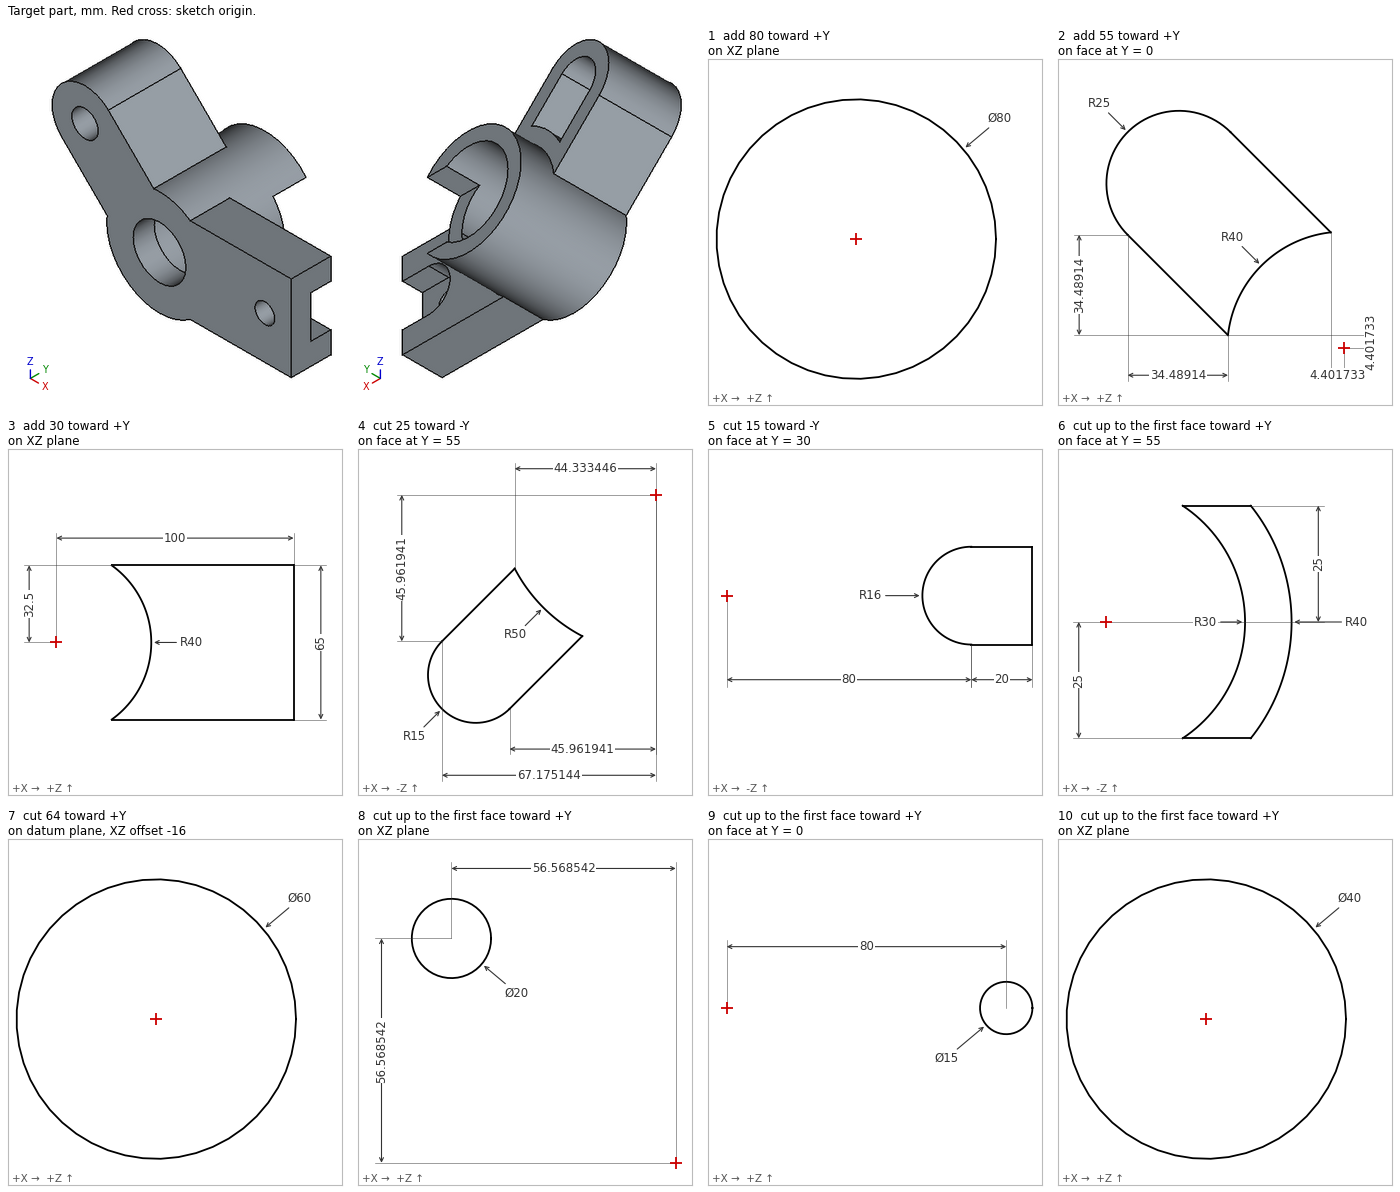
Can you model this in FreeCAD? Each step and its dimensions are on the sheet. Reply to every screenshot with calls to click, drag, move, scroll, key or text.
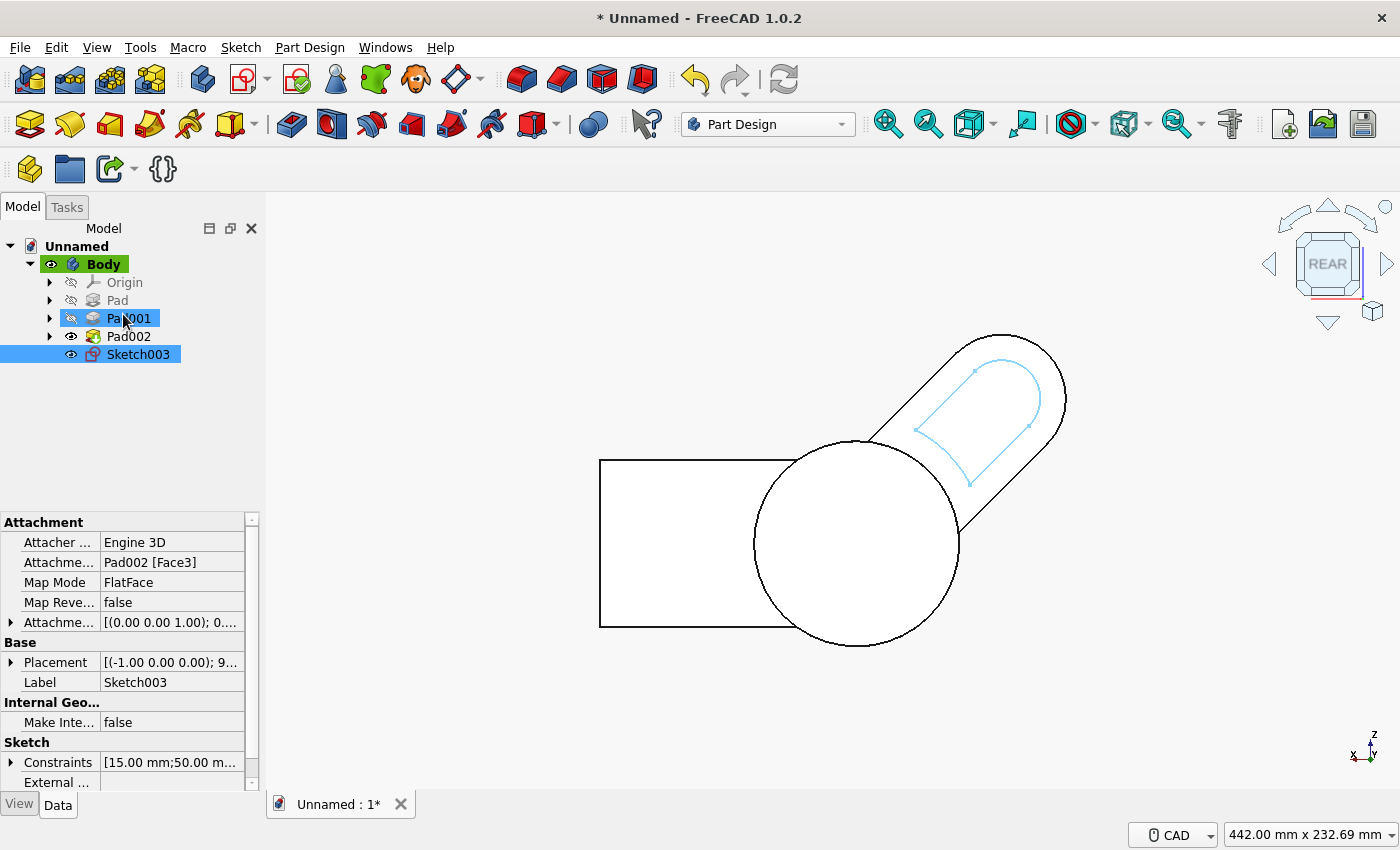
click(292, 124)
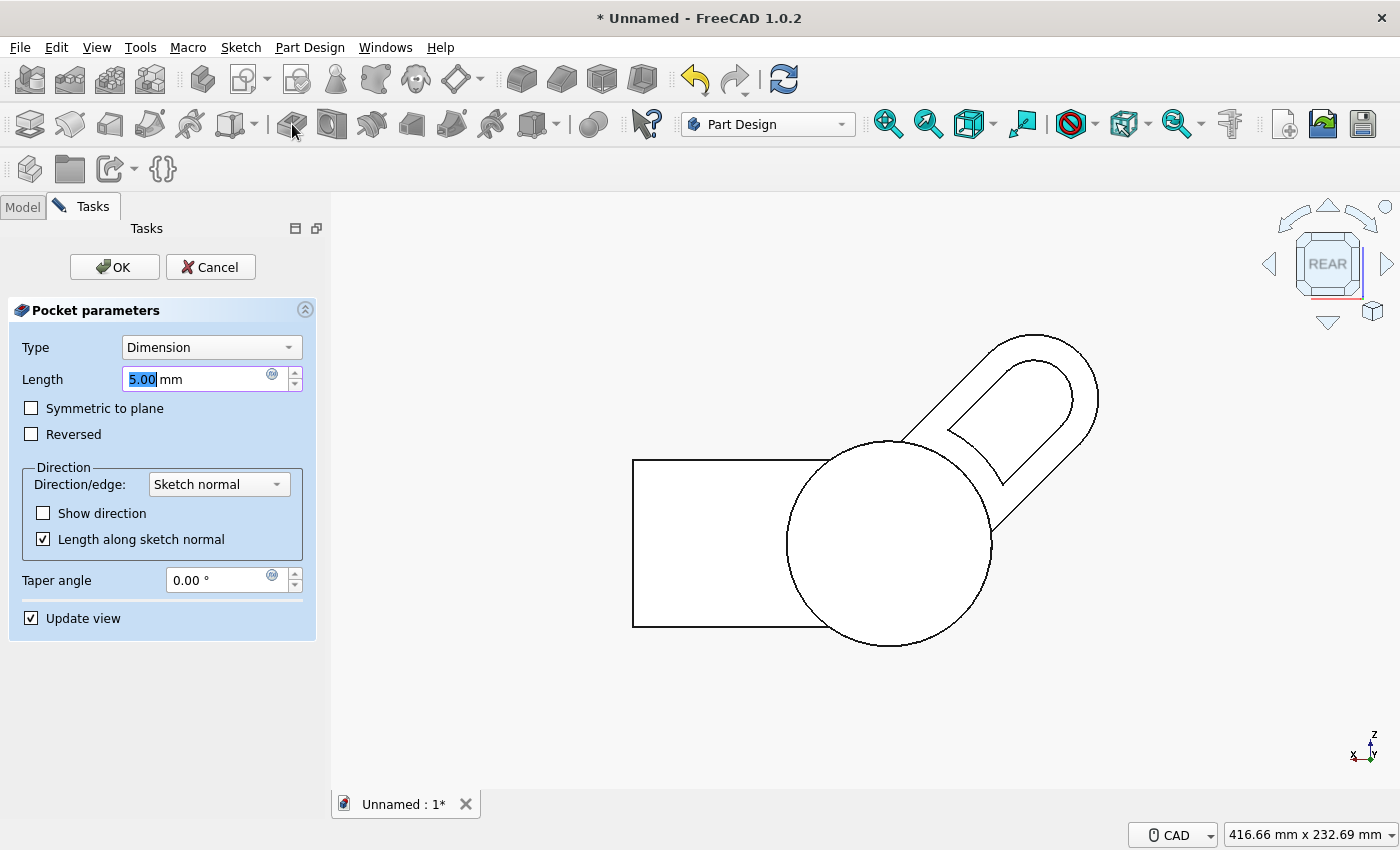
text(25)
key(Tab)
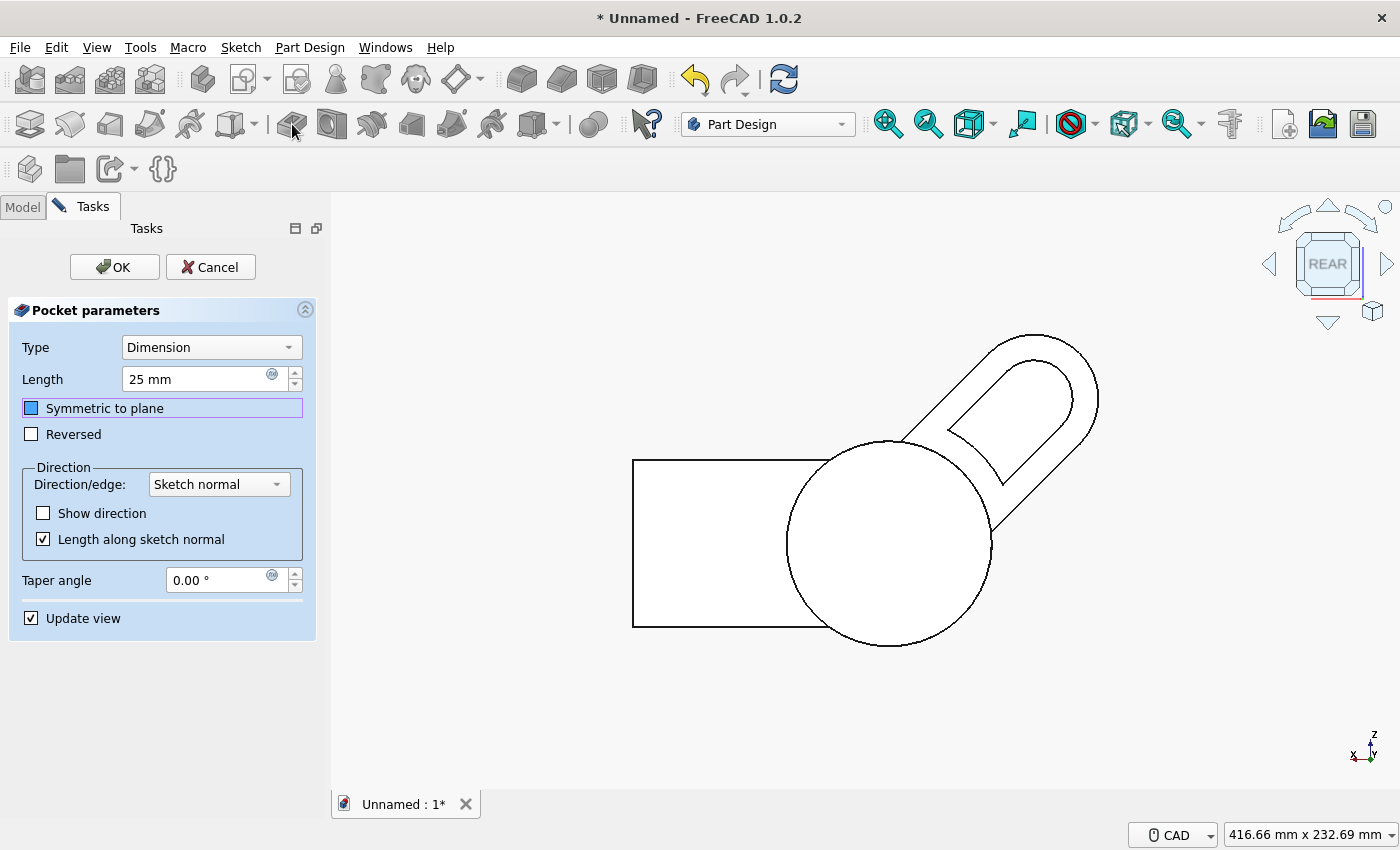
click(115, 267)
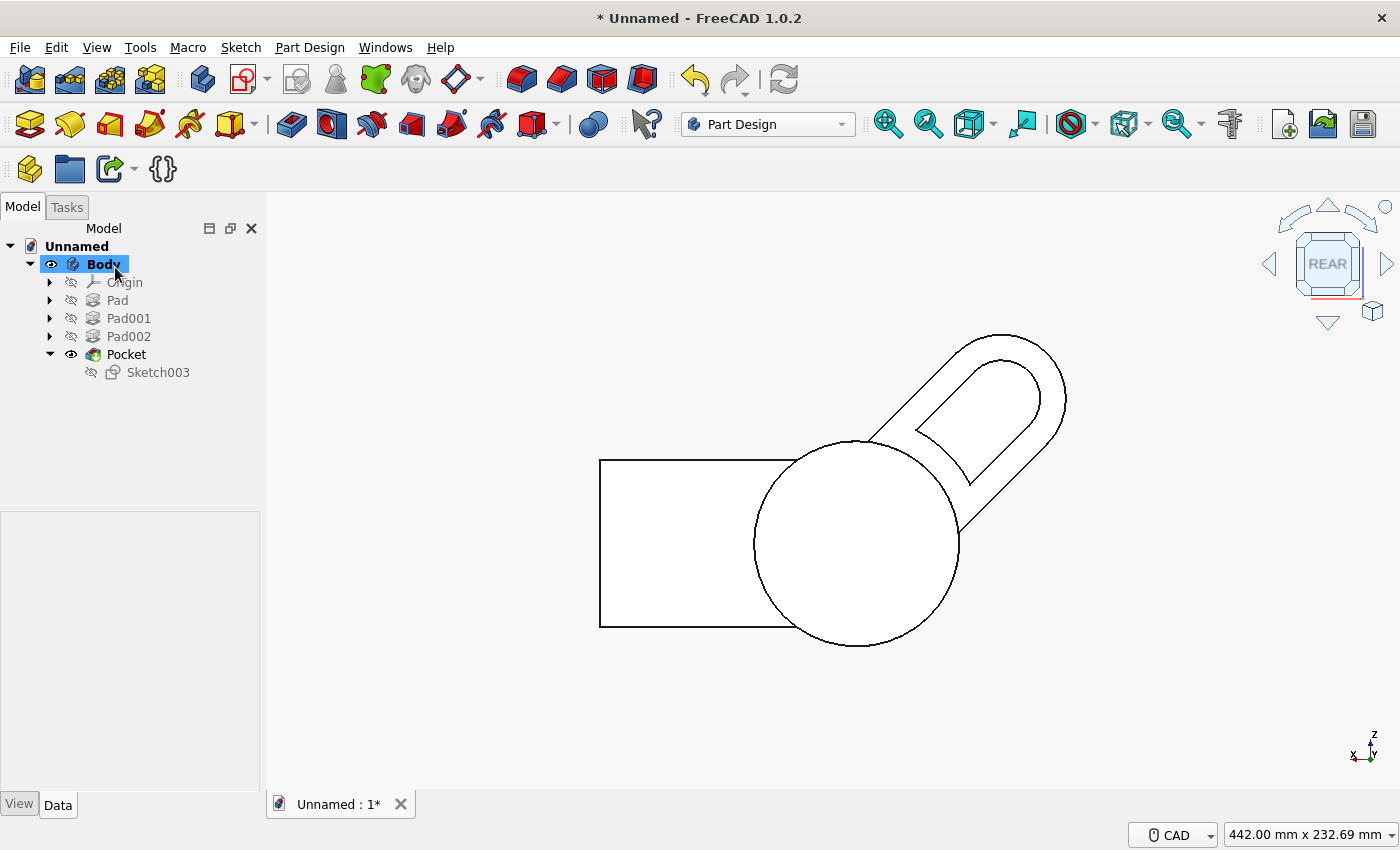
click(670, 543)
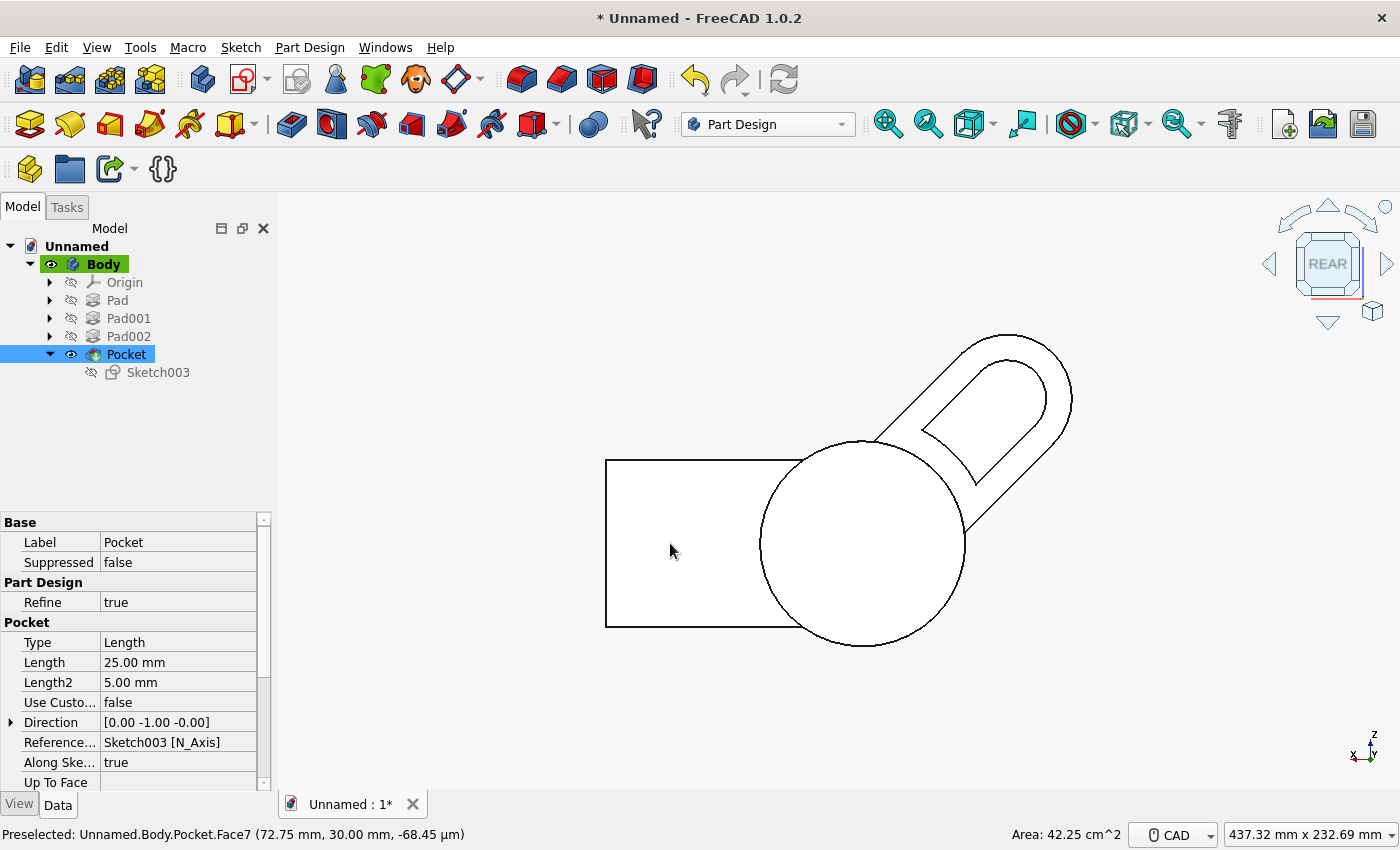
click(244, 80)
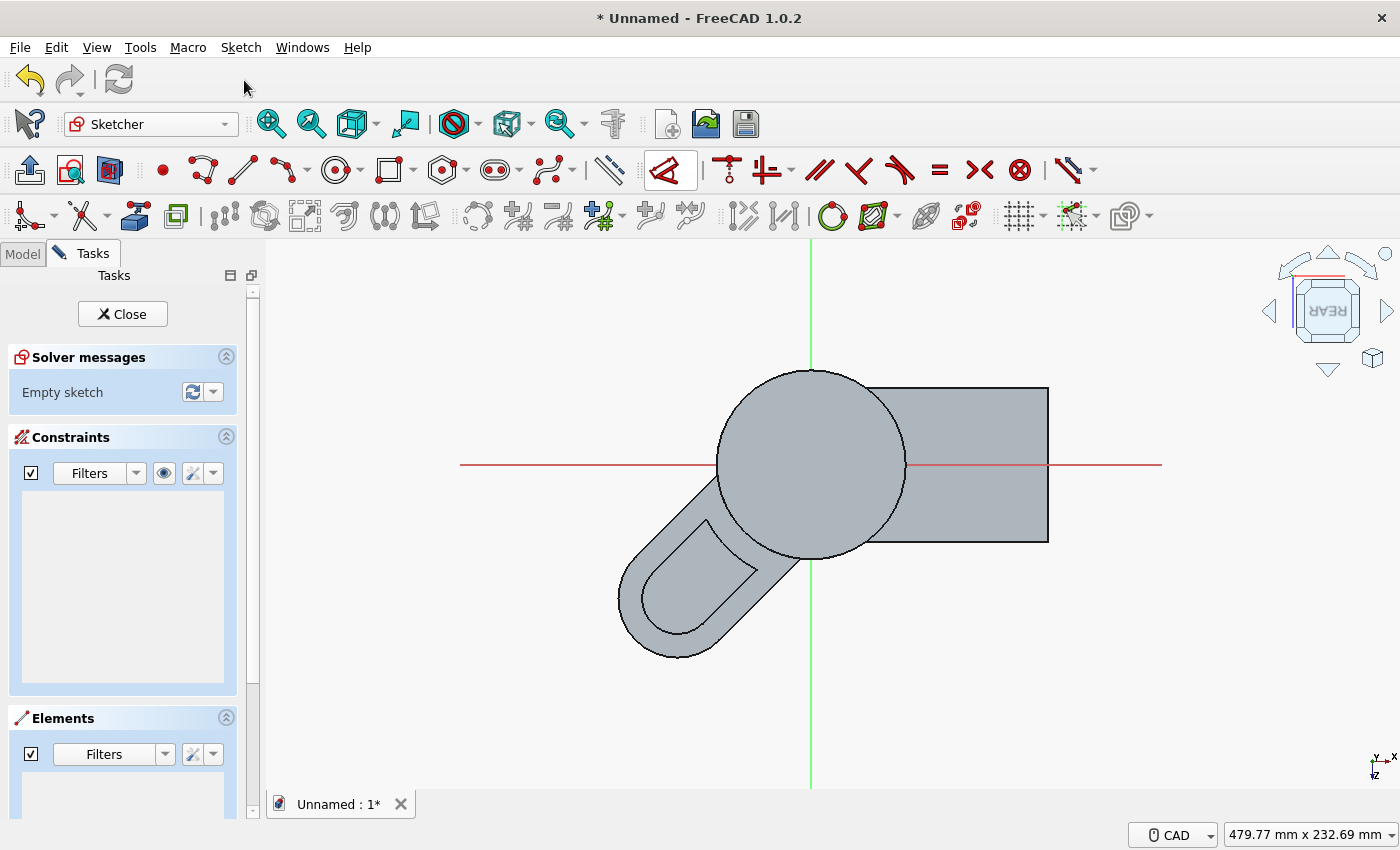
click(110, 170)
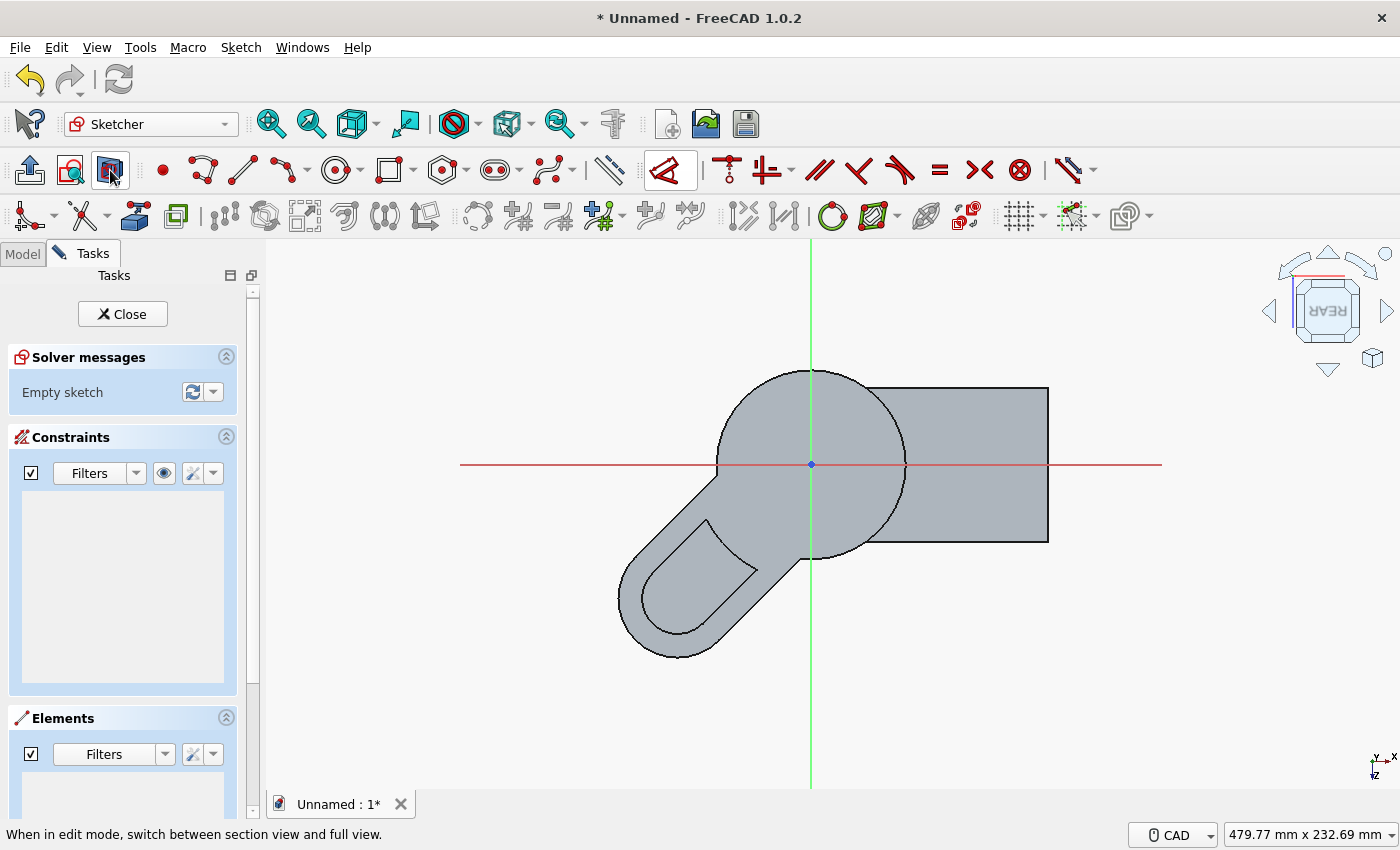
scroll(1066, 452, up, 8)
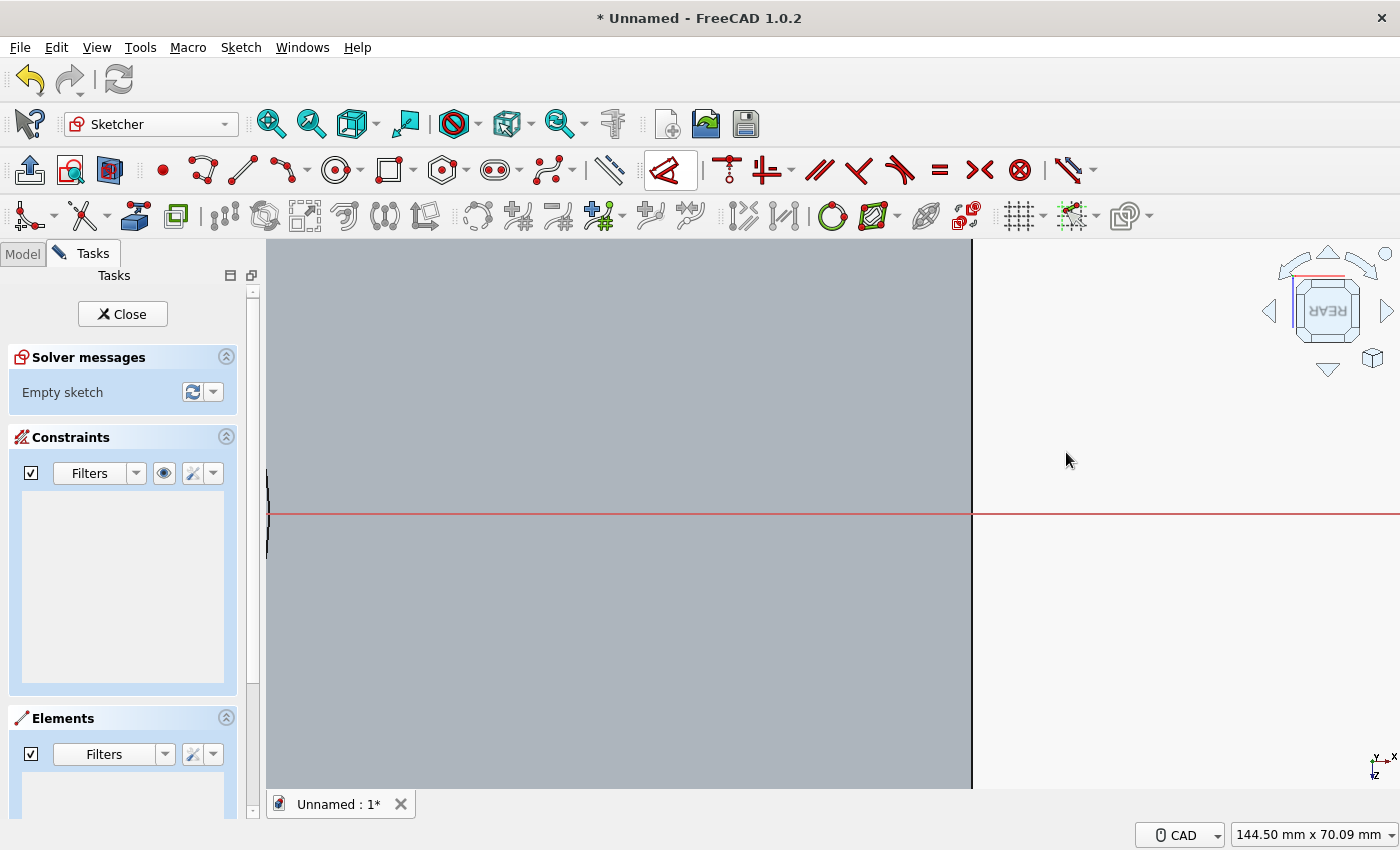
click(204, 170)